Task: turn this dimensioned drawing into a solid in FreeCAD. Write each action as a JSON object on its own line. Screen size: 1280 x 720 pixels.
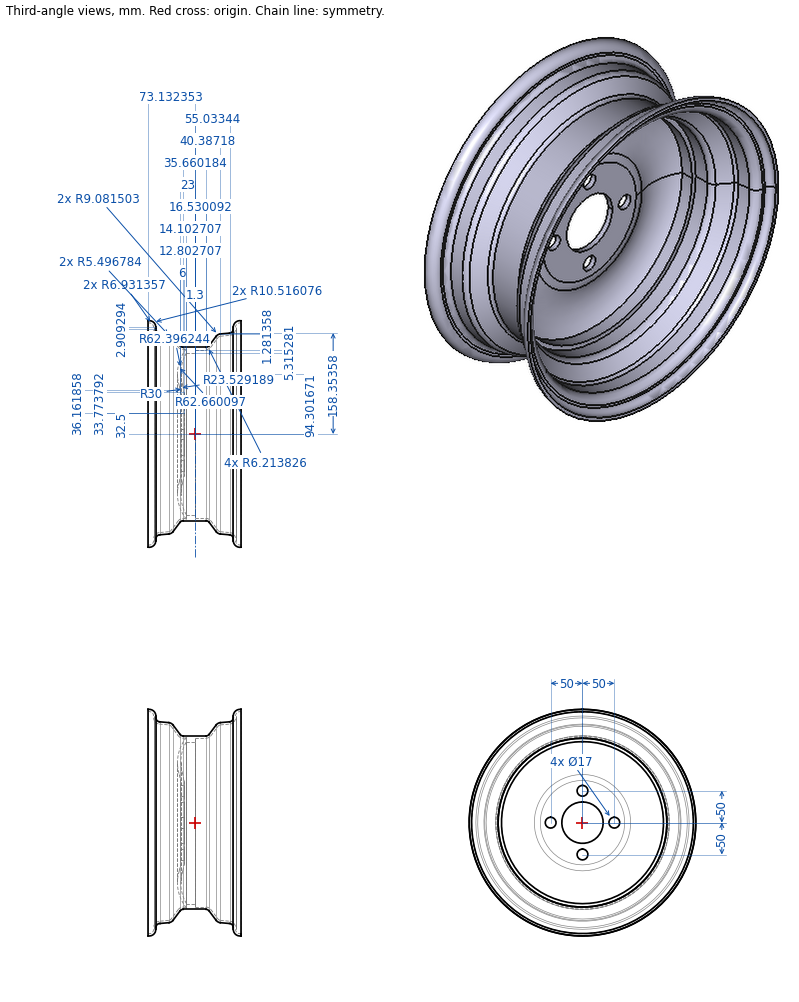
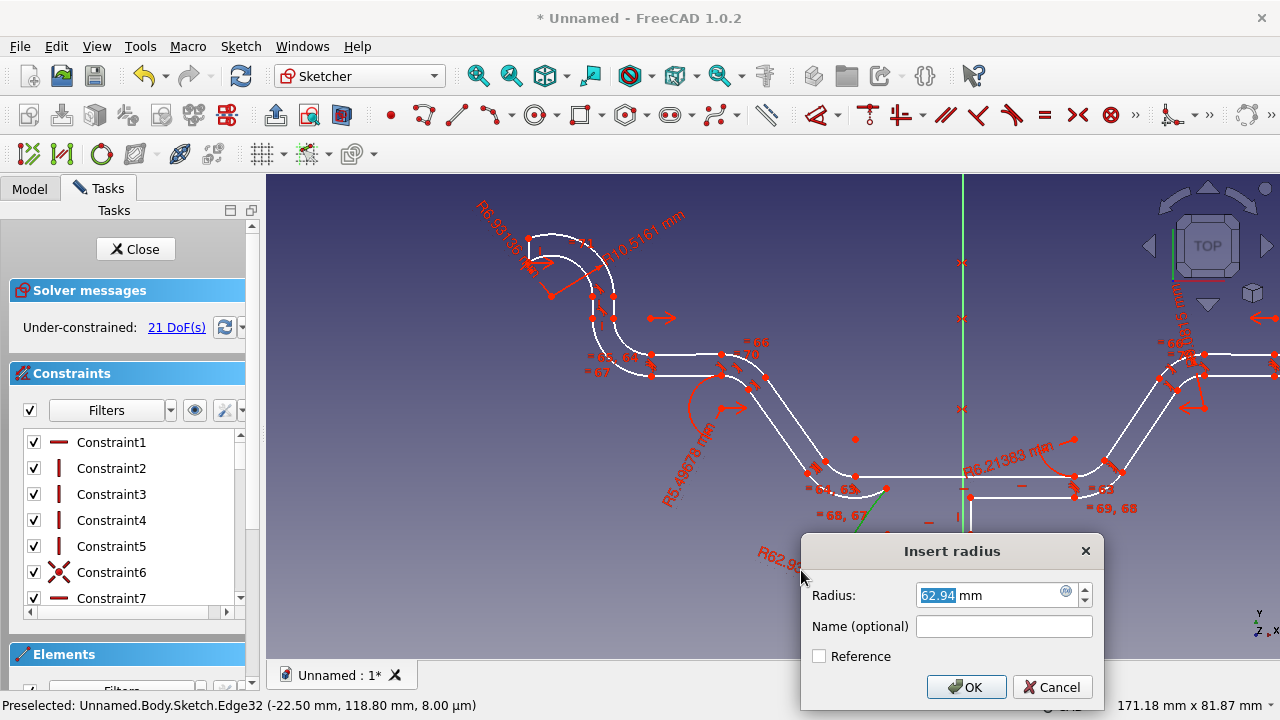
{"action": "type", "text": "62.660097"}
{"action": "key", "text": "Return"}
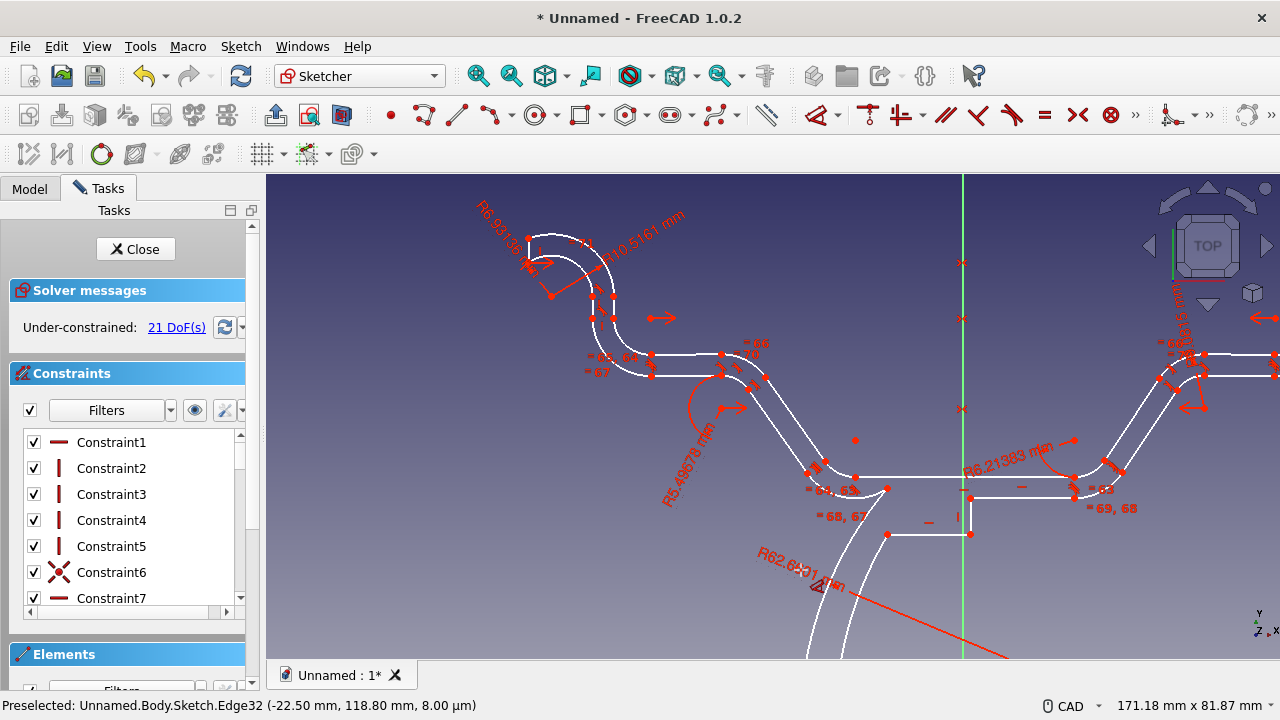
{"action": "scroll", "coordinate": [593, 269], "scroll_direction": "down", "scroll_amount": 6}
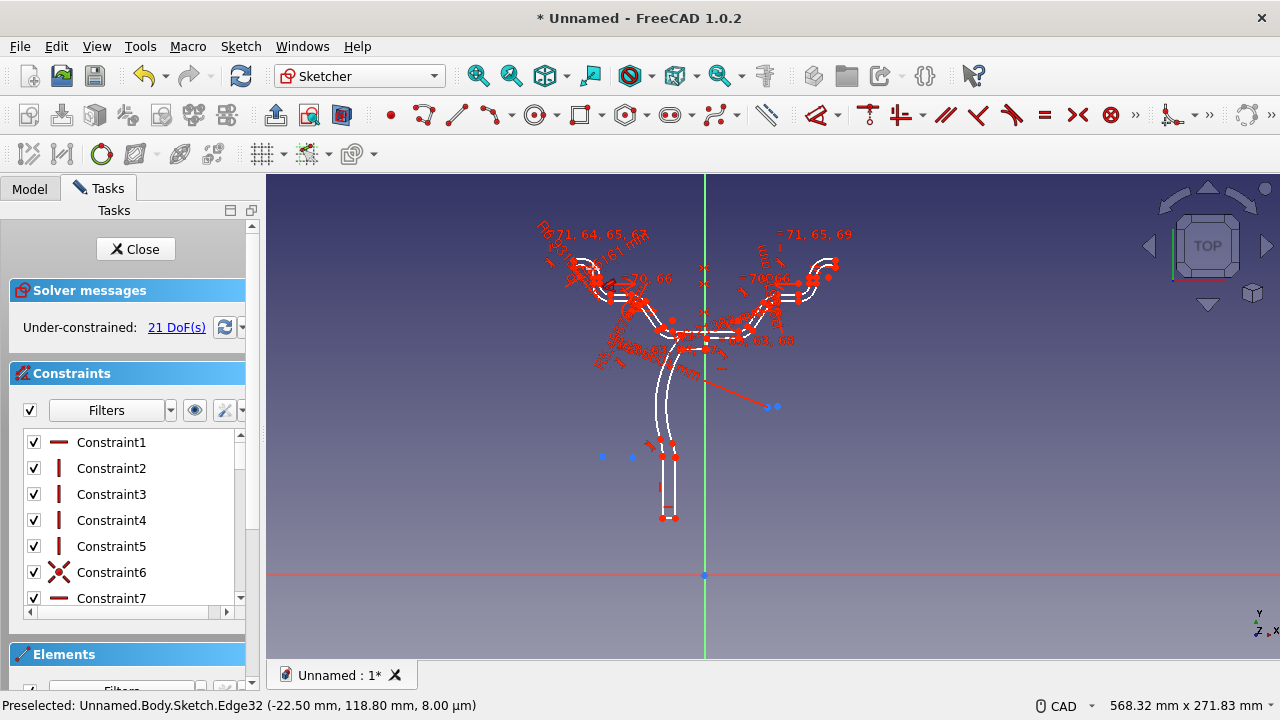
{"action": "scroll", "coordinate": [663, 451], "scroll_direction": "up", "scroll_amount": 5}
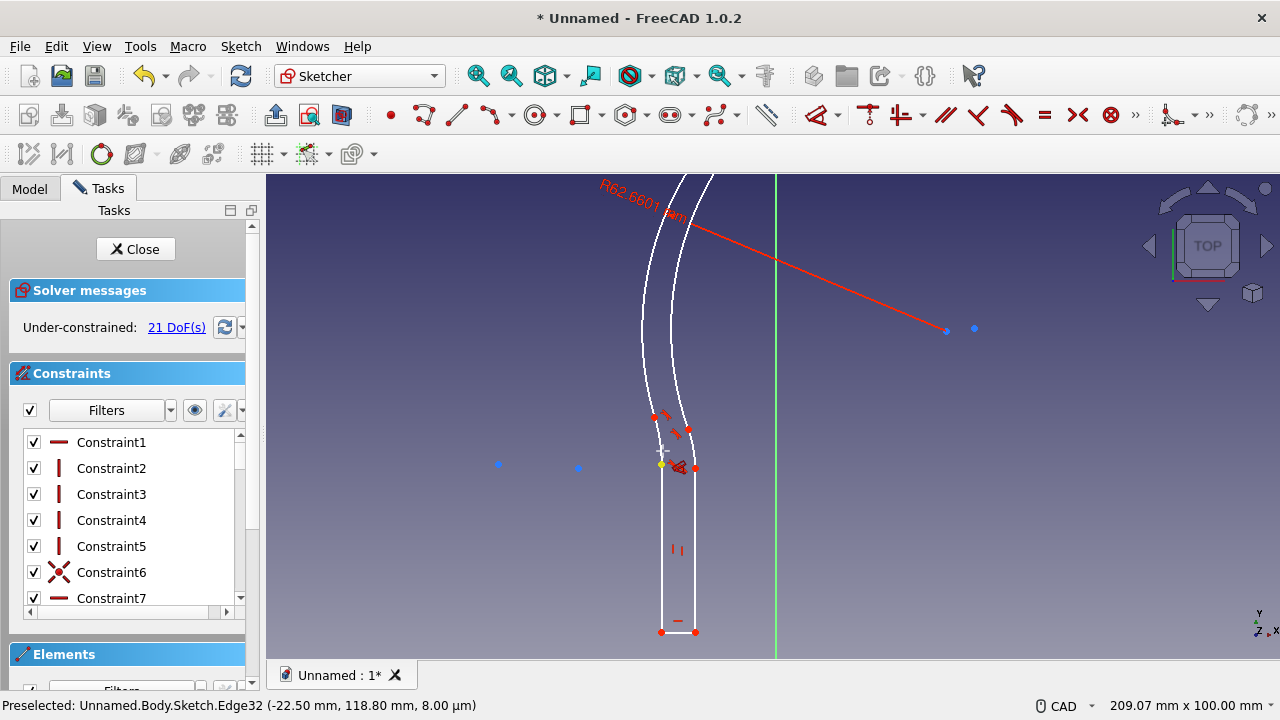
{"action": "left_click", "coordinate": [661, 450]}
{"action": "left_click", "coordinate": [677, 543]}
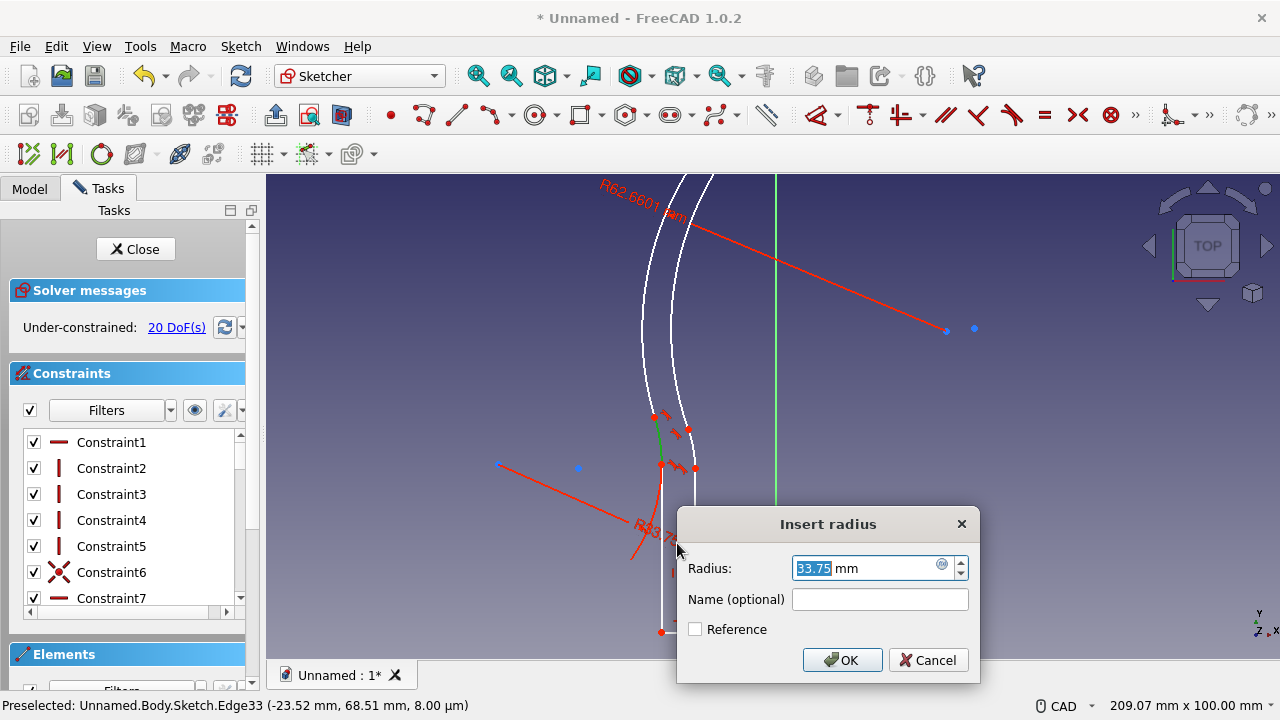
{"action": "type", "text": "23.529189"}
{"action": "key", "text": "Return"}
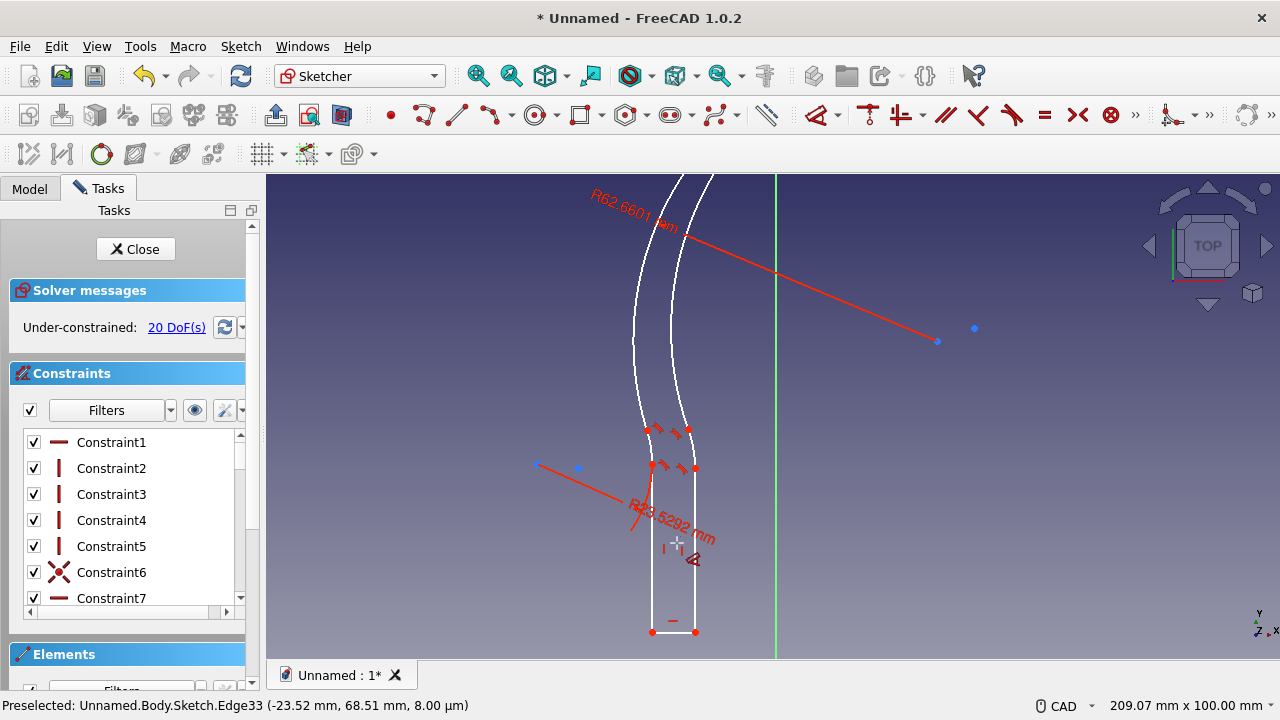
{"action": "left_click", "coordinate": [694, 457]}
{"action": "left_click", "coordinate": [726, 454]}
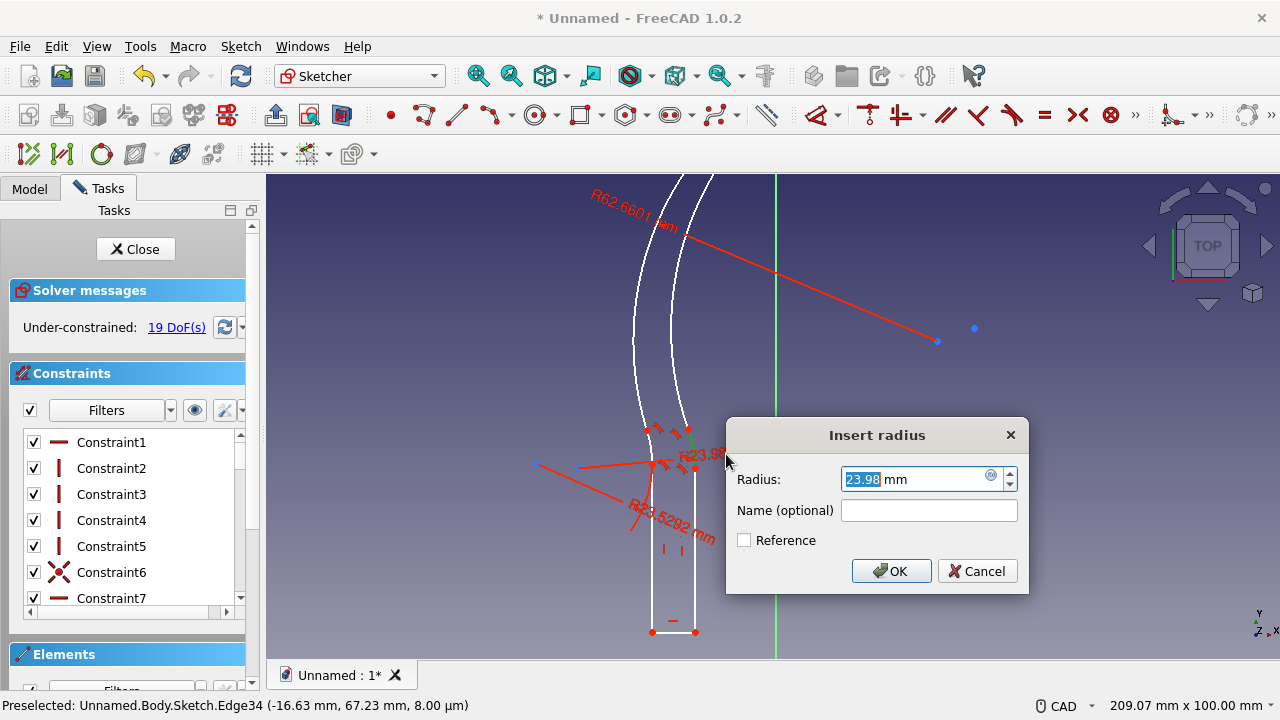
{"action": "type", "text": "30"}
{"action": "key", "text": "Return"}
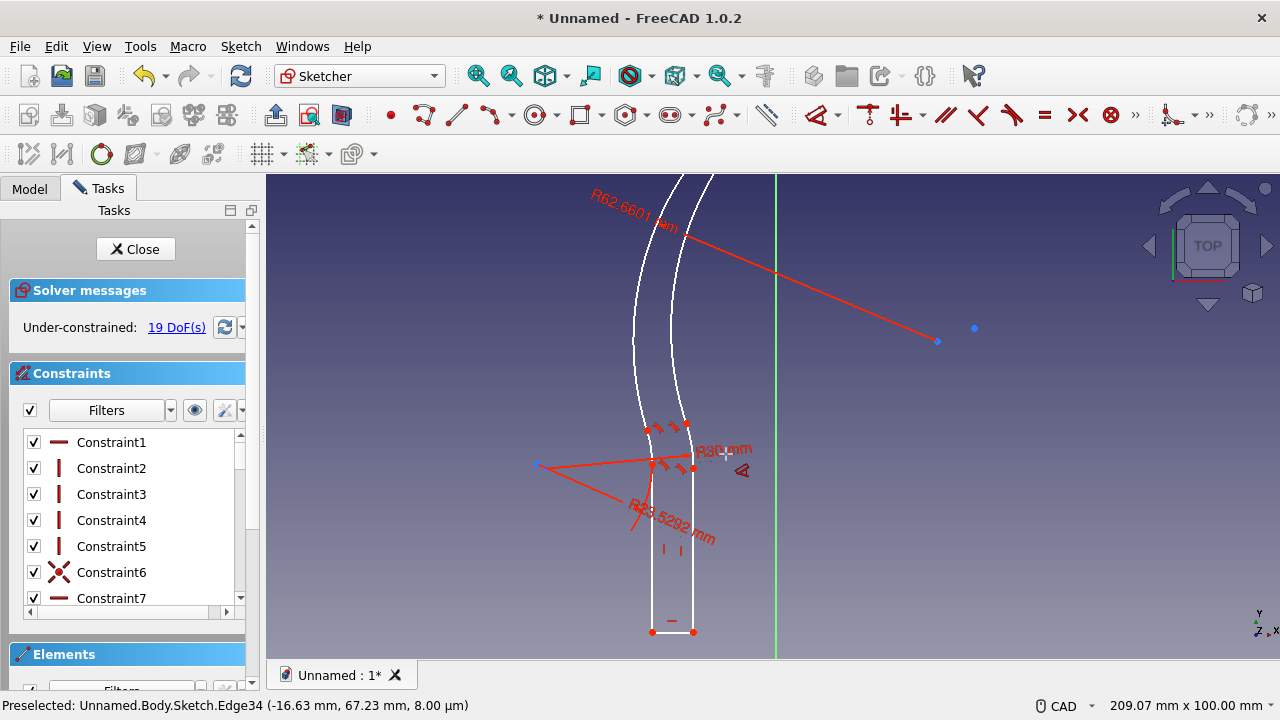
{"action": "left_click", "coordinate": [683, 244]}
{"action": "left_click", "coordinate": [630, 229]}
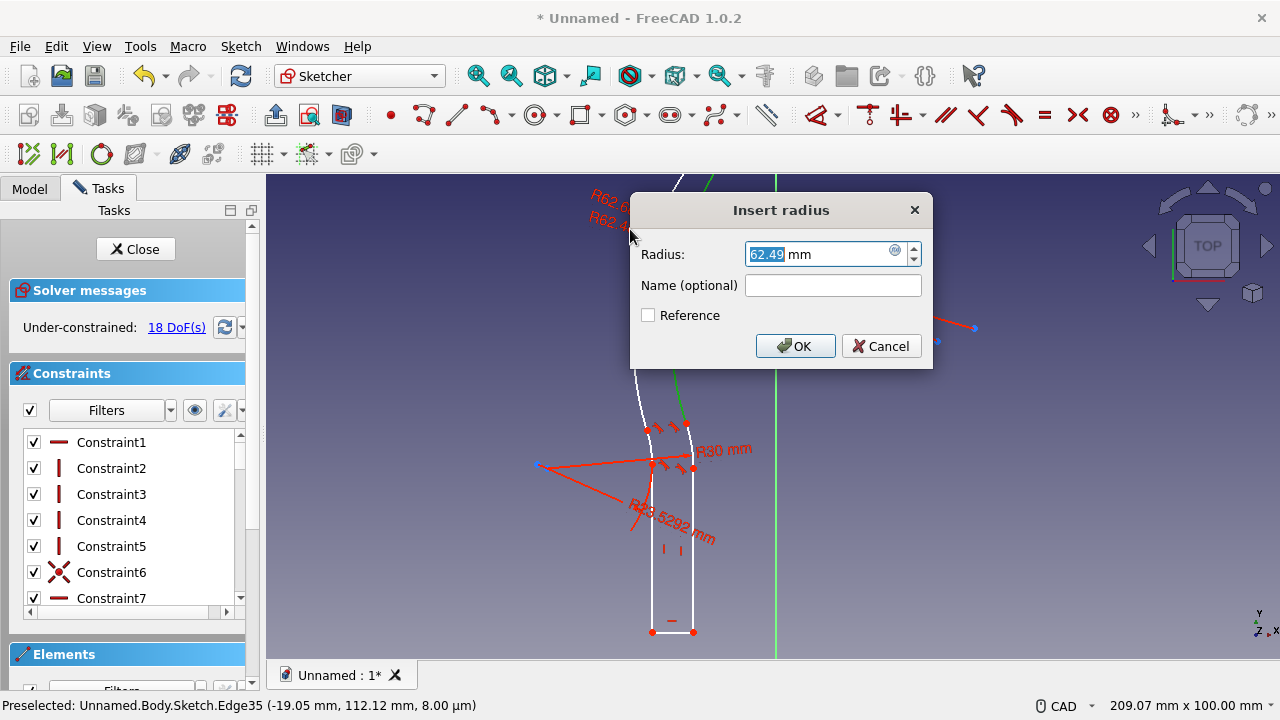
{"action": "type", "text": "62.396244"}
{"action": "key", "text": "Return"}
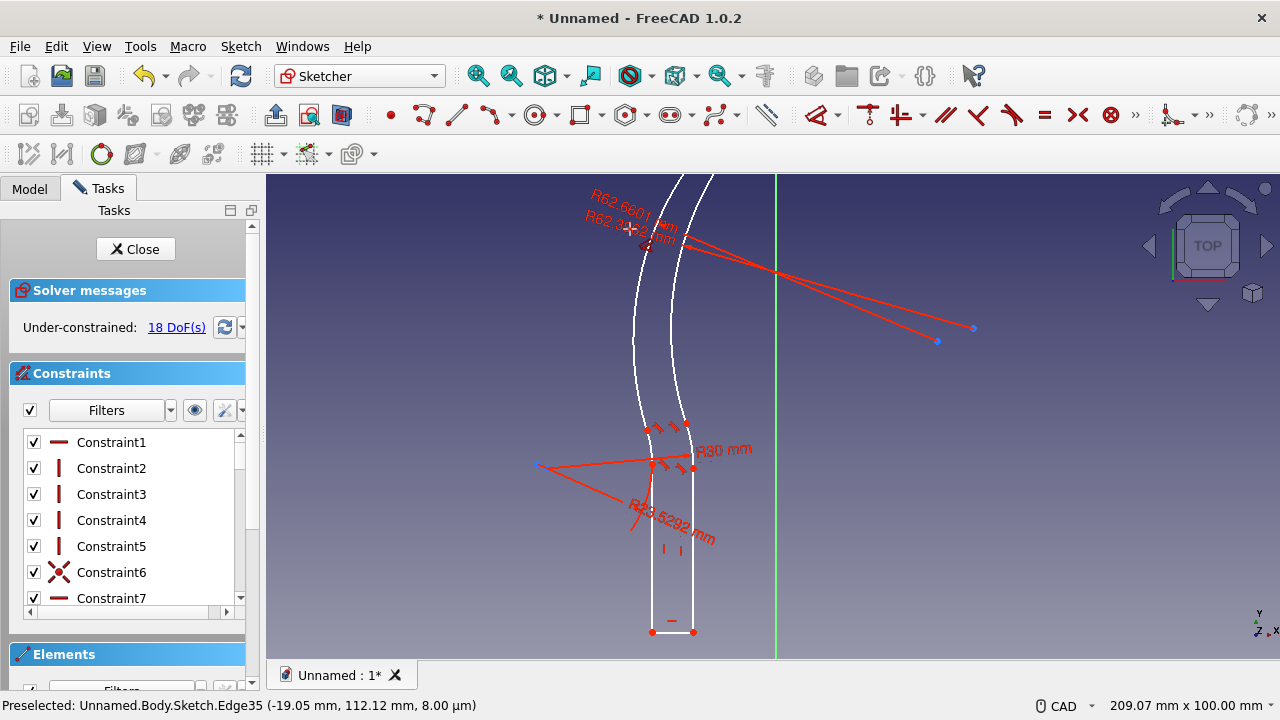
{"action": "scroll", "coordinate": [663, 451], "scroll_direction": "down", "scroll_amount": 5}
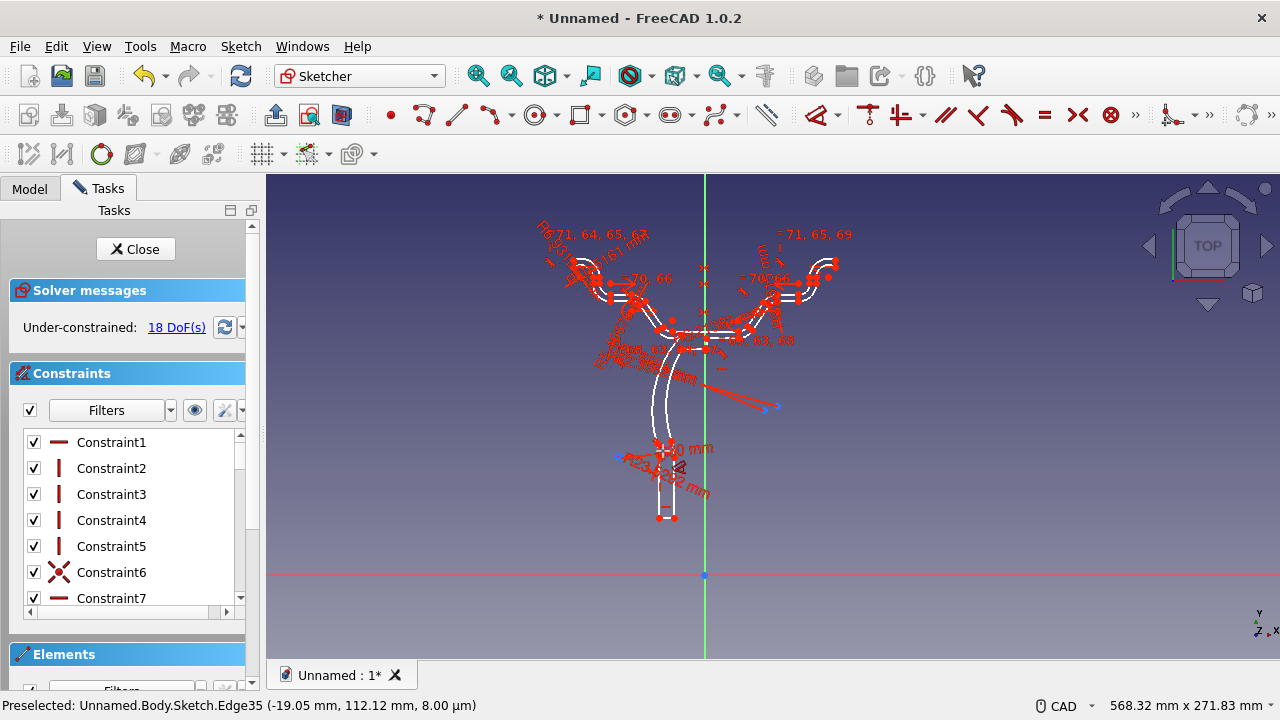
{"action": "scroll", "coordinate": [664, 518], "scroll_direction": "up", "scroll_amount": 7}